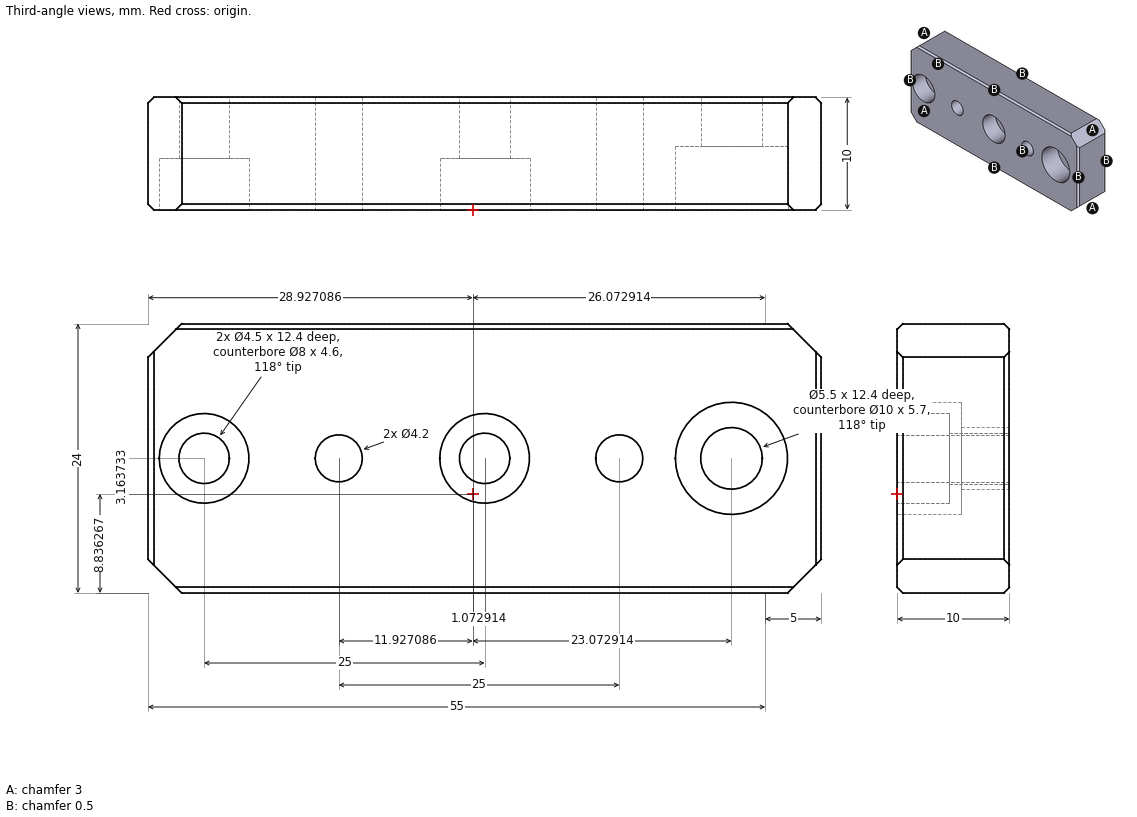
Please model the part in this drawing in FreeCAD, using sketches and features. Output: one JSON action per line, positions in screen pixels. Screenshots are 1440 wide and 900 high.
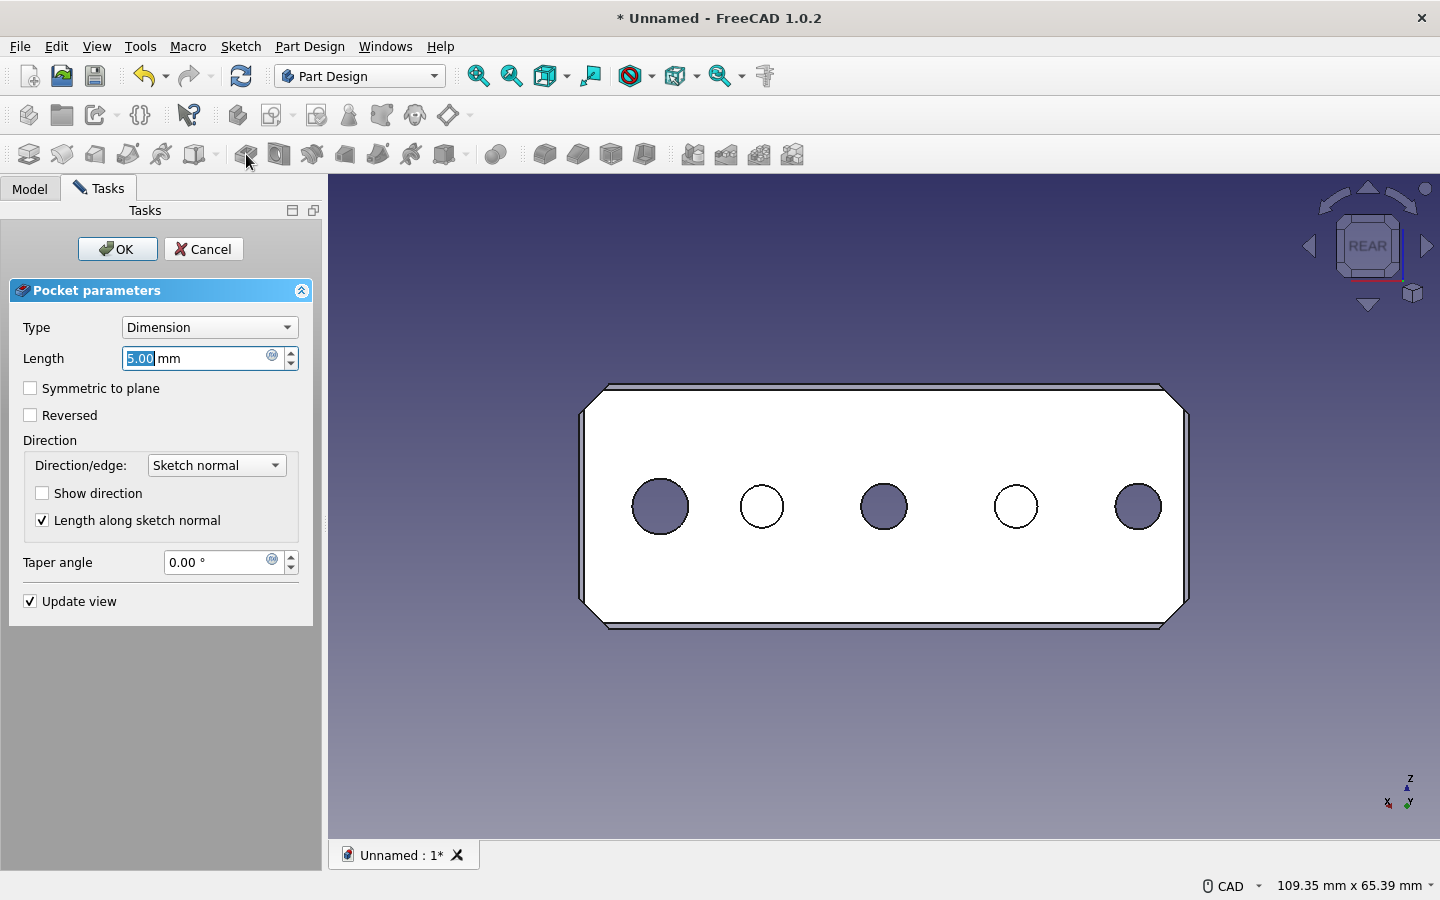
{"action": "left_click", "coordinate": [210, 328]}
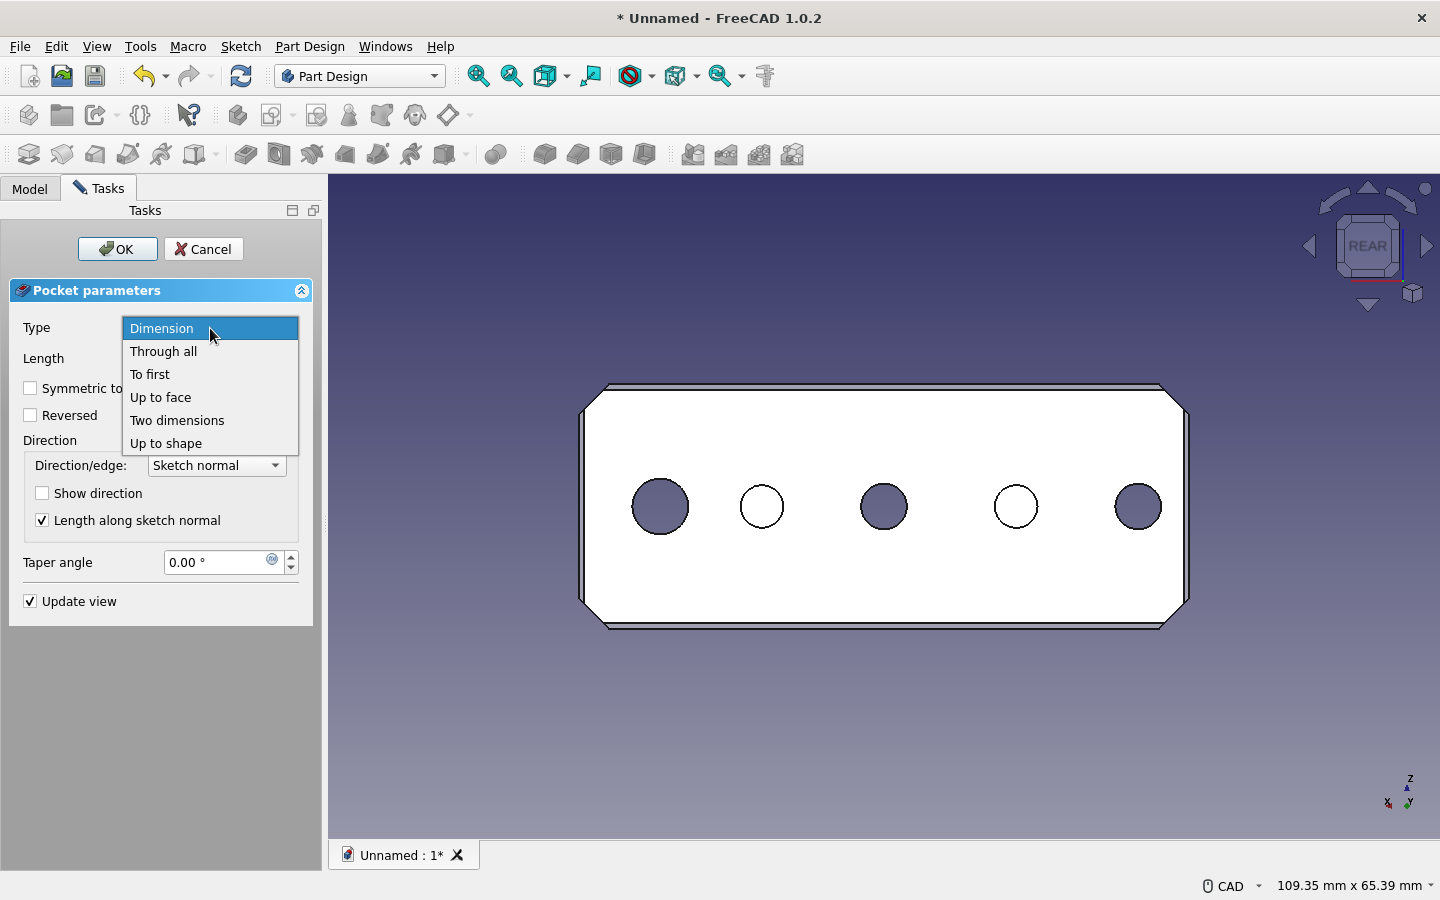
{"action": "left_click", "coordinate": [208, 352]}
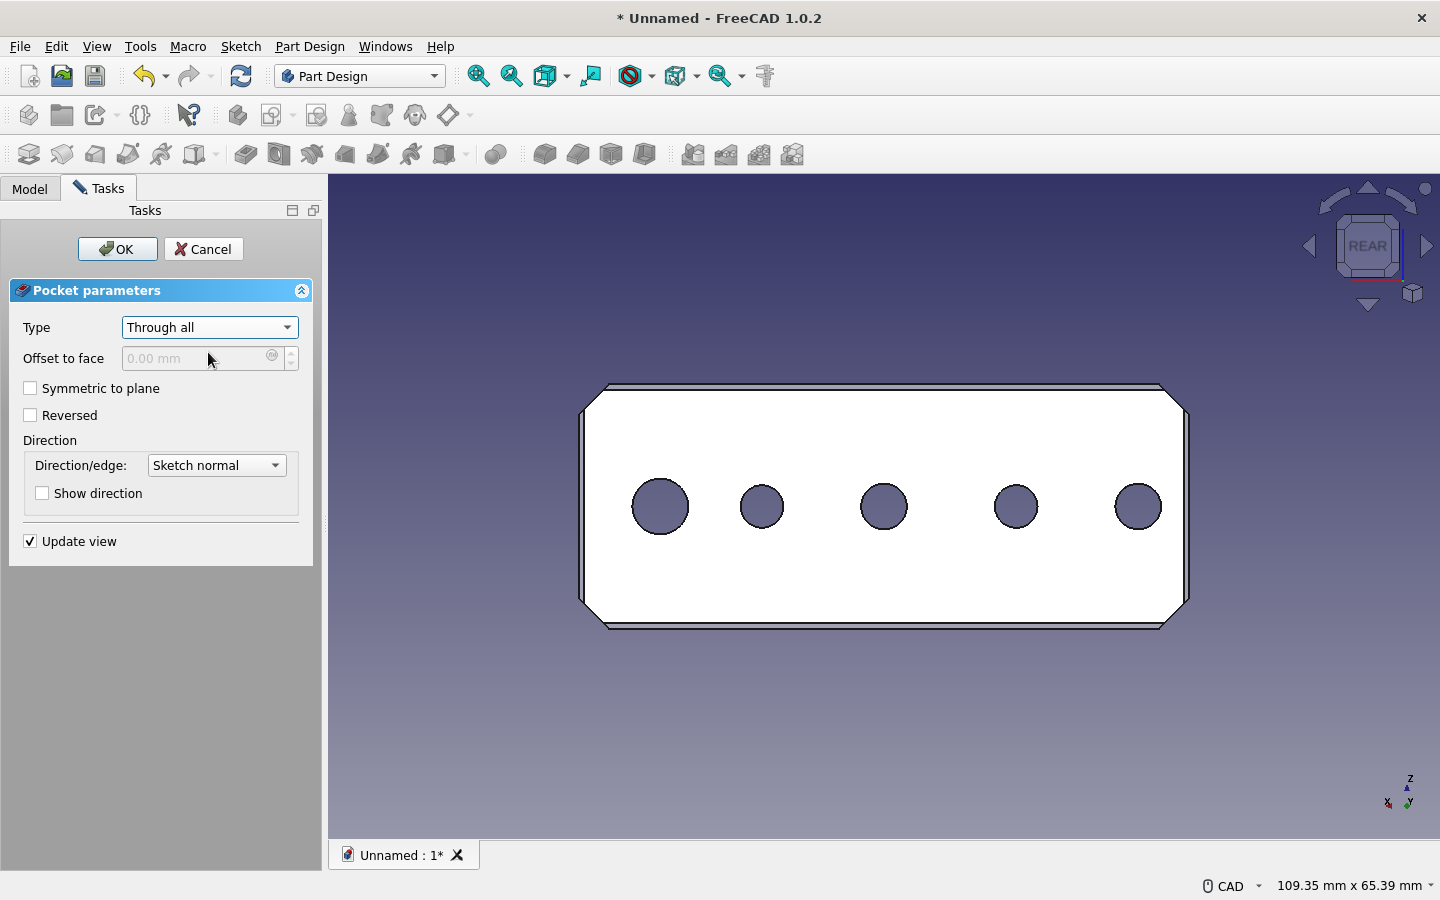
{"action": "left_click", "coordinate": [118, 249]}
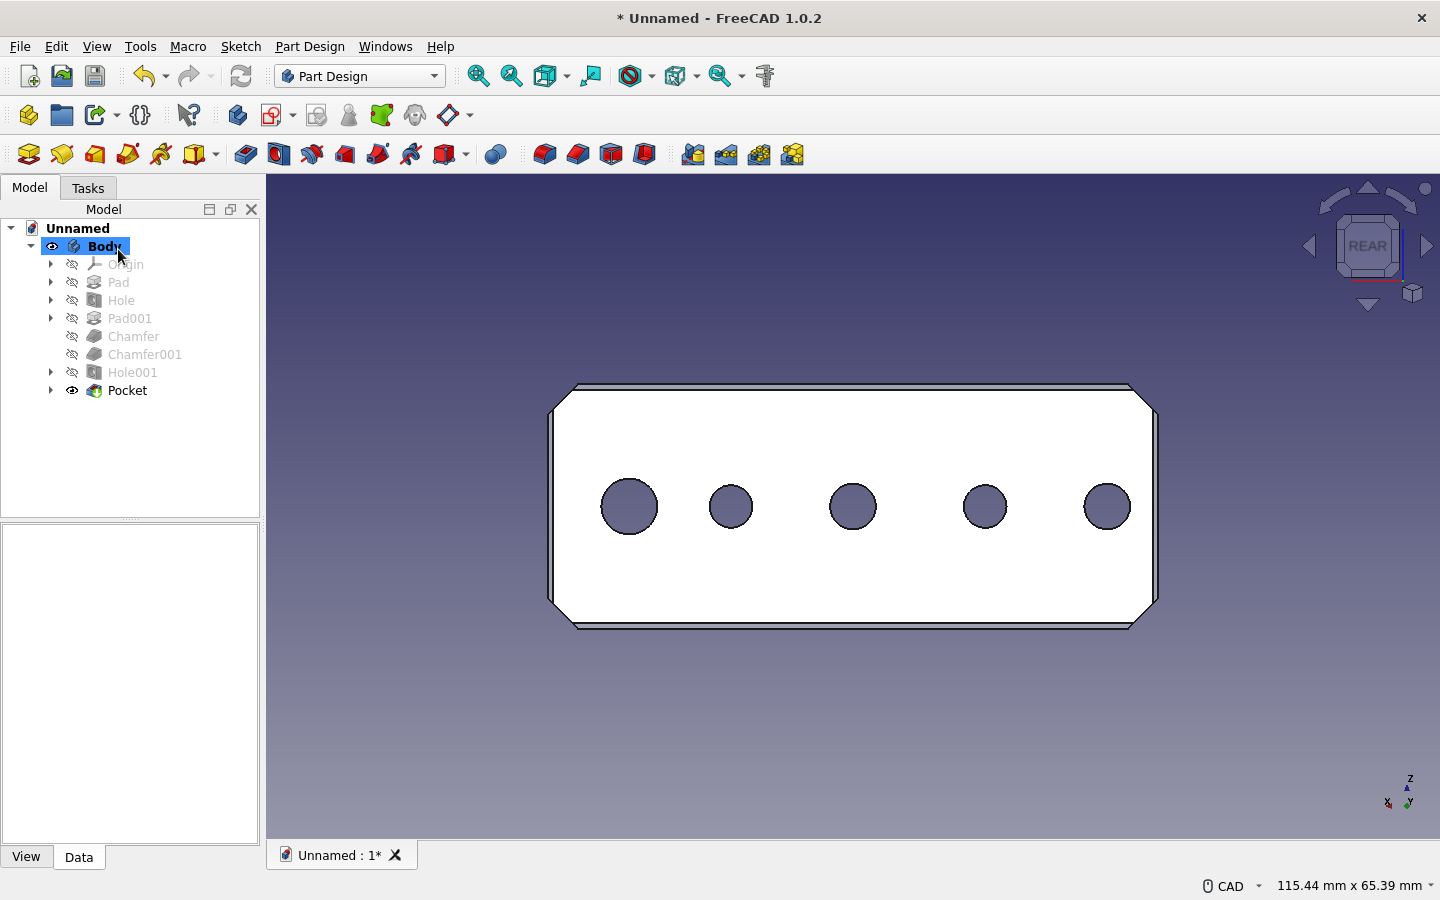
{"action": "key", "text": "0"}